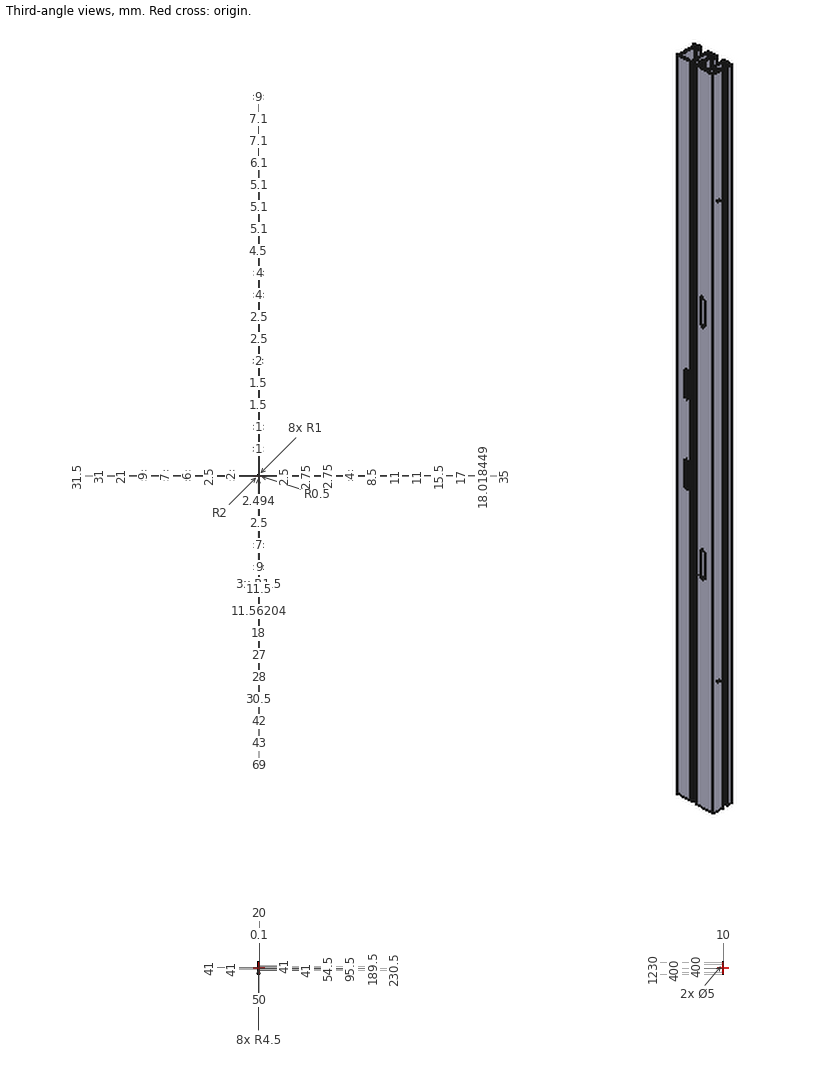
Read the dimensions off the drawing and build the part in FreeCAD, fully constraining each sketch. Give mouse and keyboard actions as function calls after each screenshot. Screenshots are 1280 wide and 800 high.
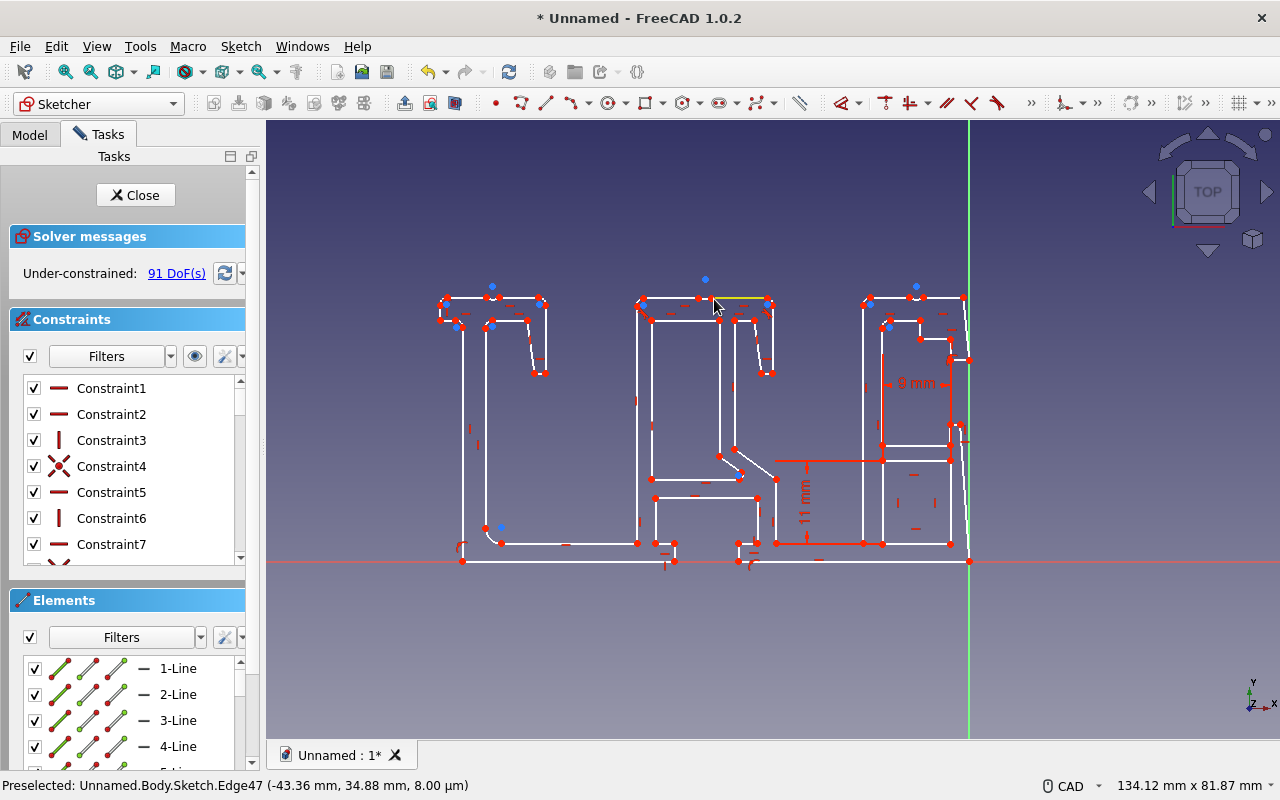
click(637, 378)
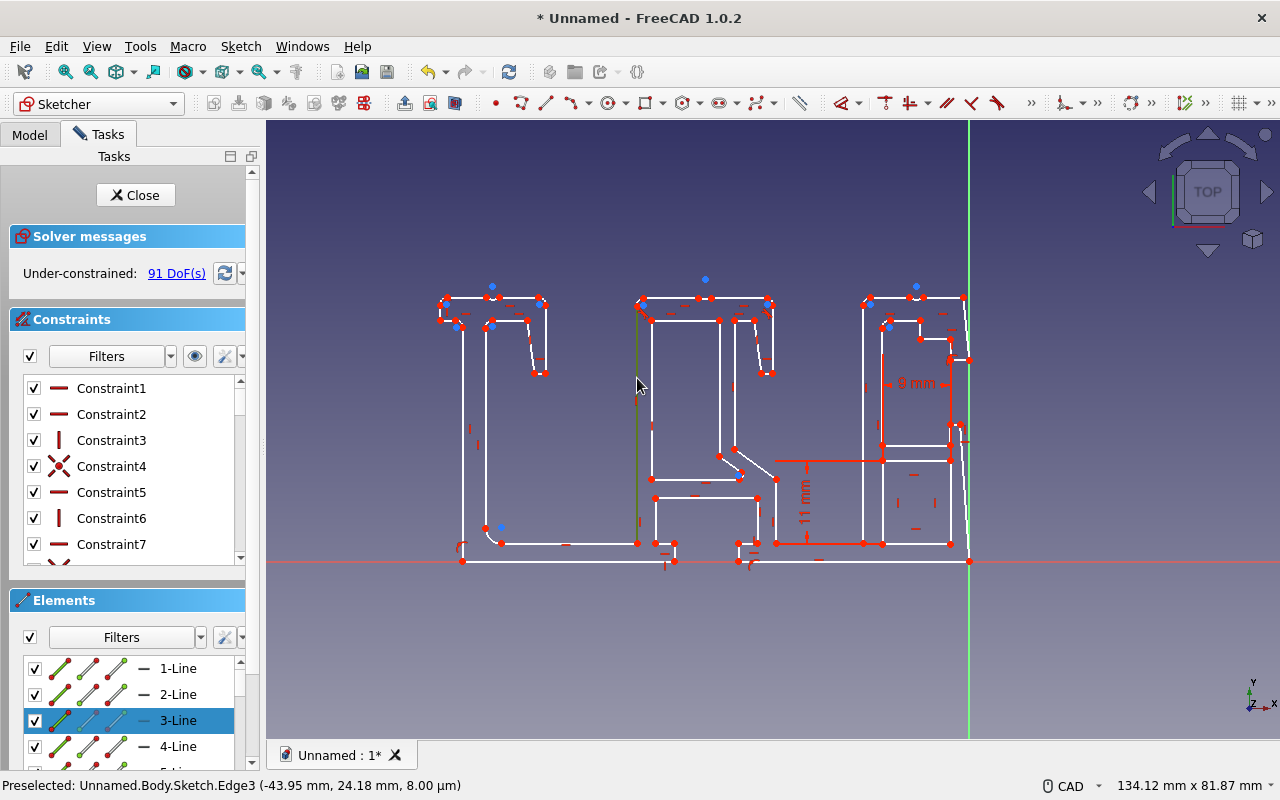
scroll(638, 301, up, 4)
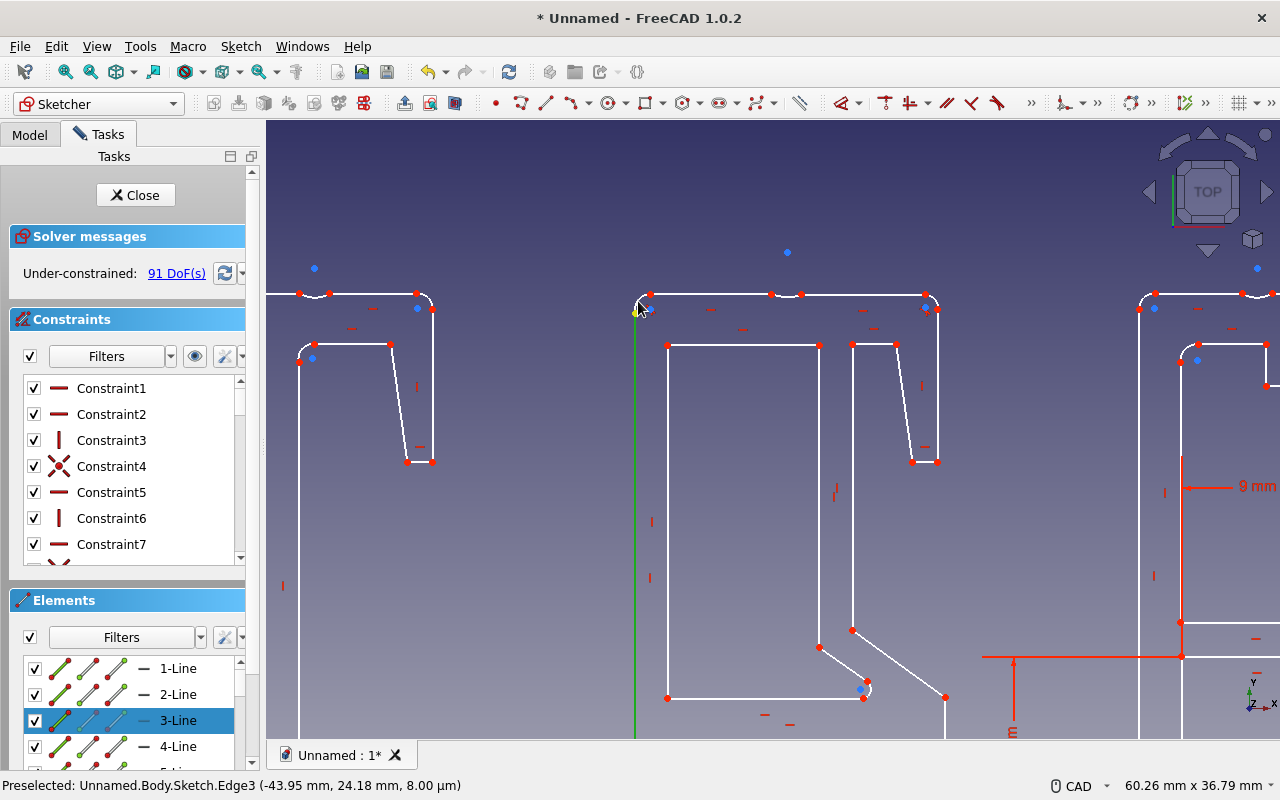
click(638, 300)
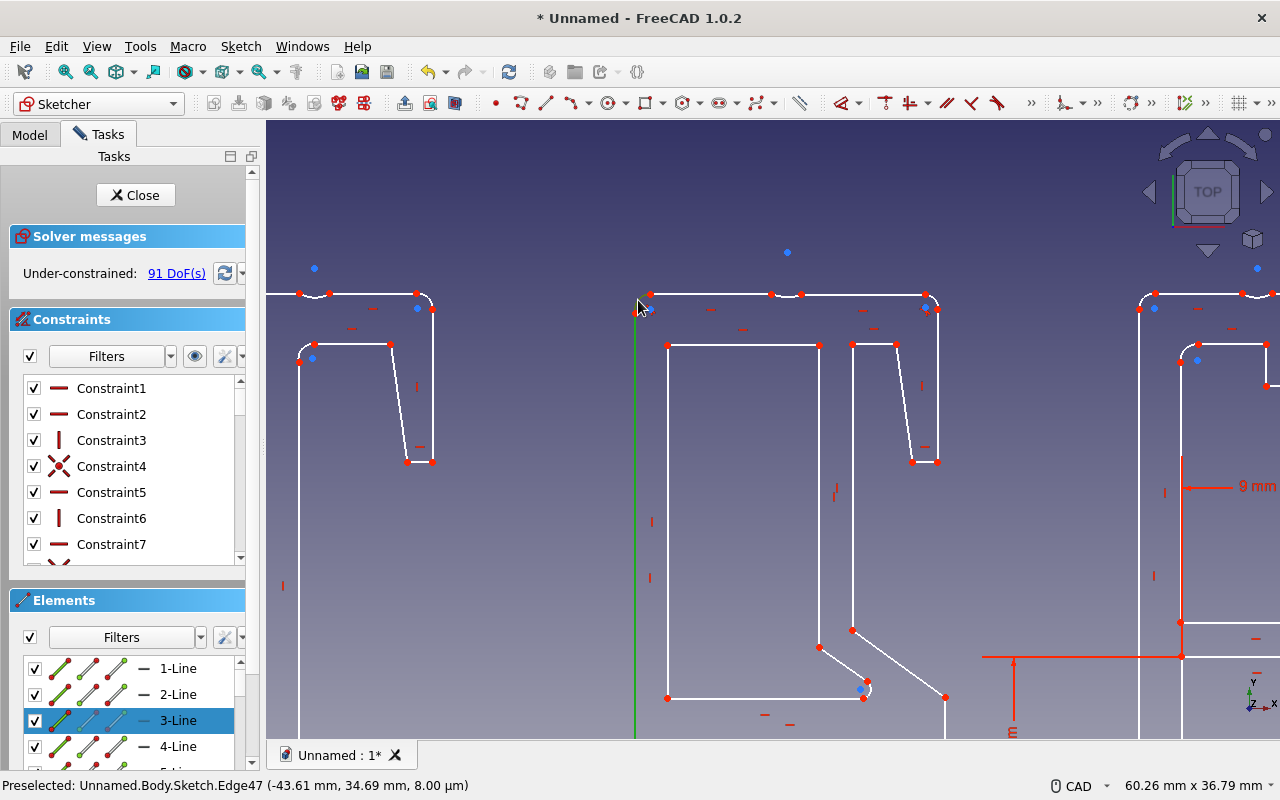
click(997, 104)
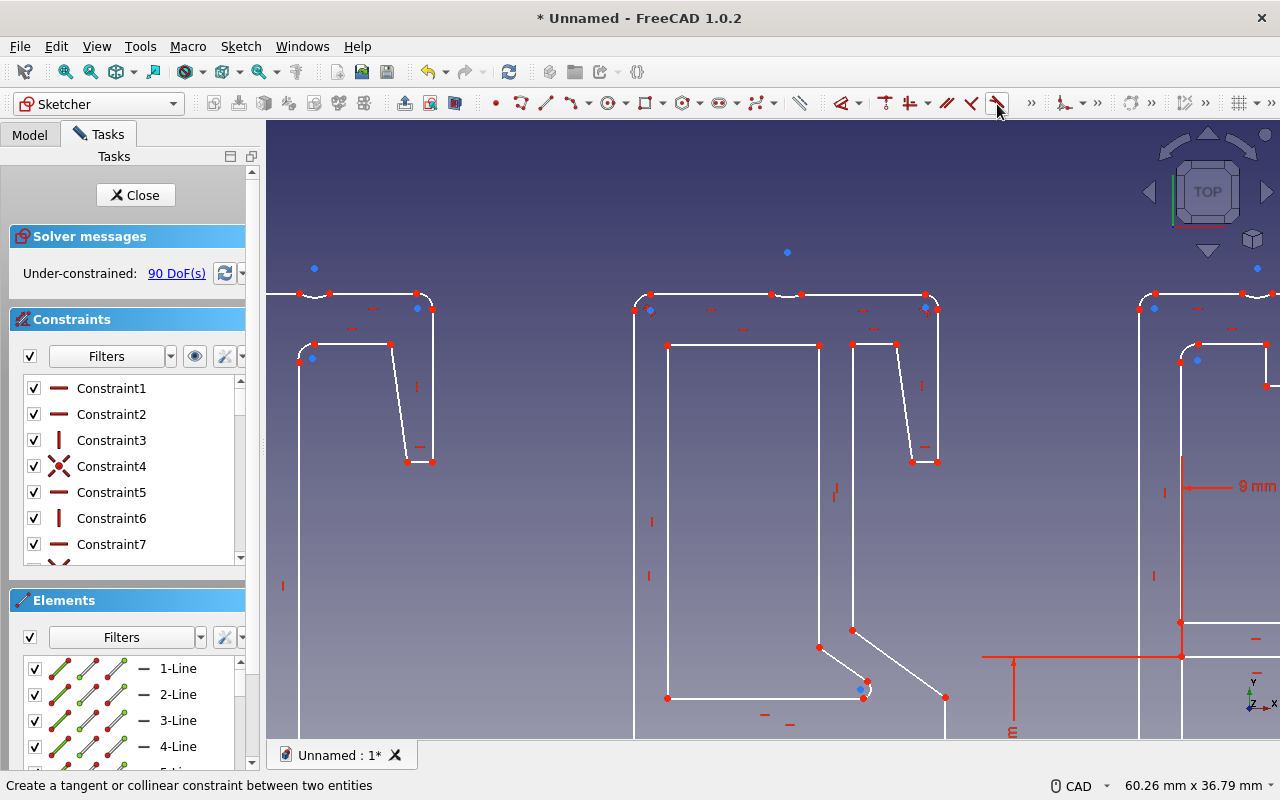
scroll(638, 301, down, 4)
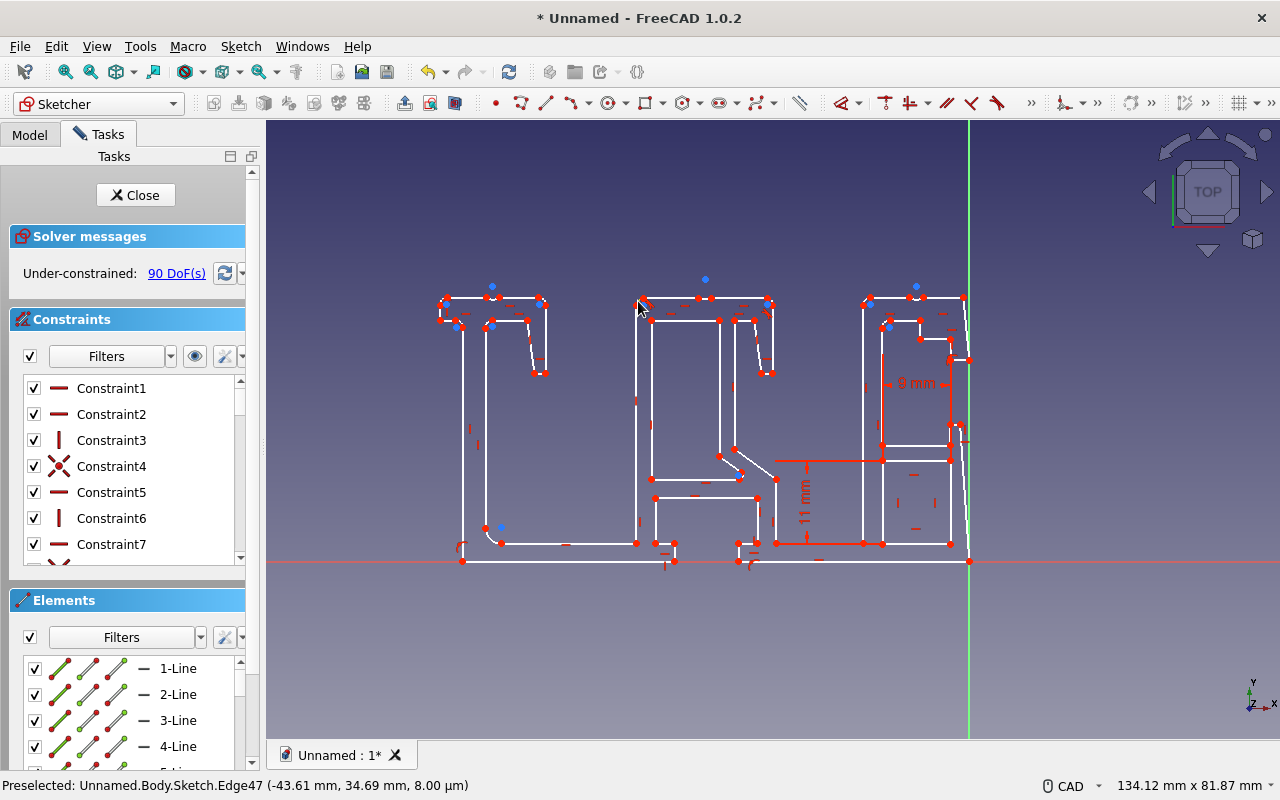
click(596, 544)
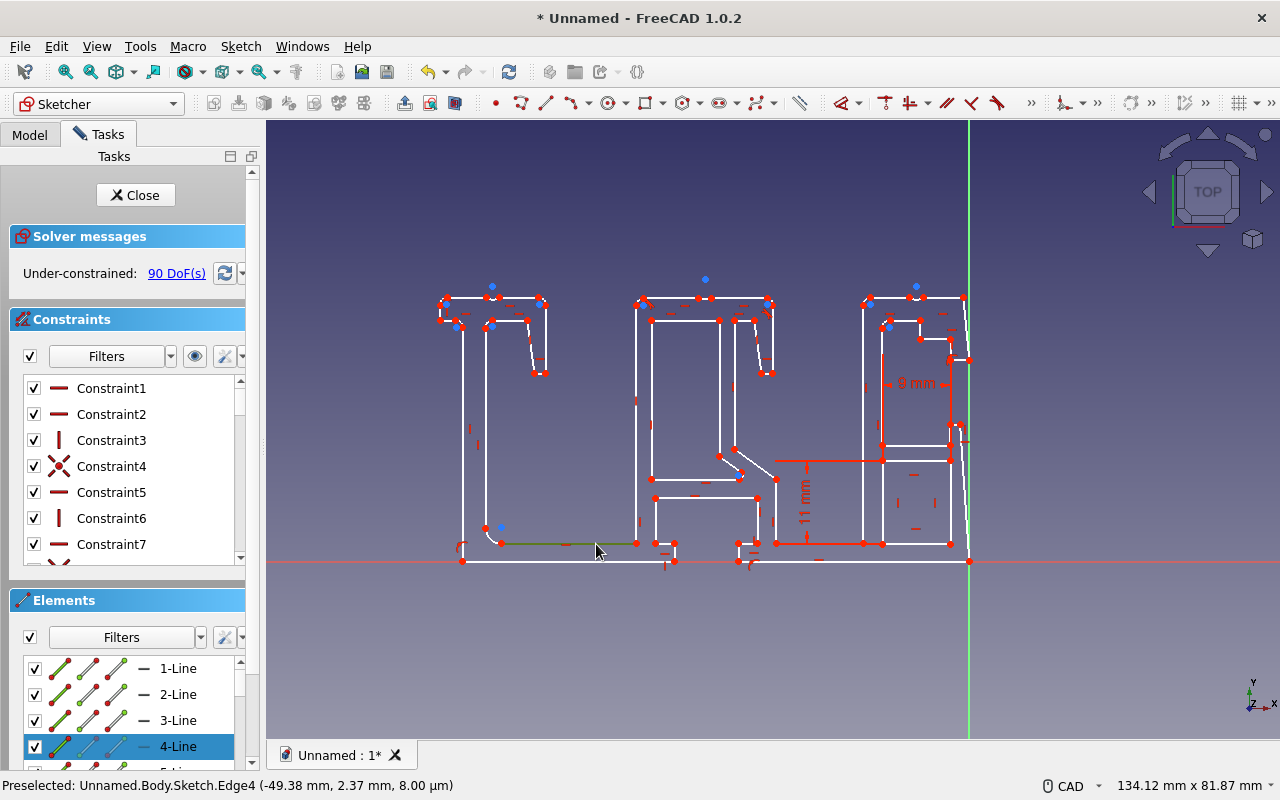
click(491, 539)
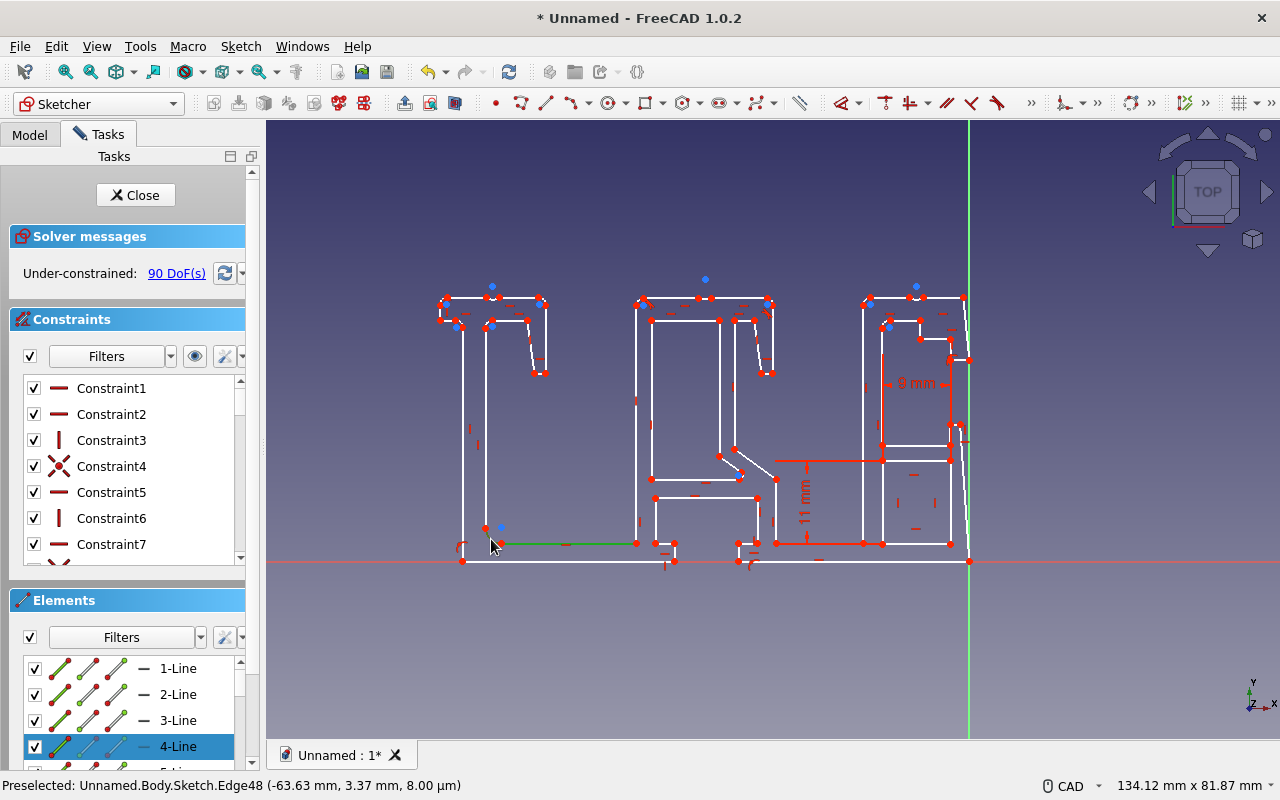
click(997, 104)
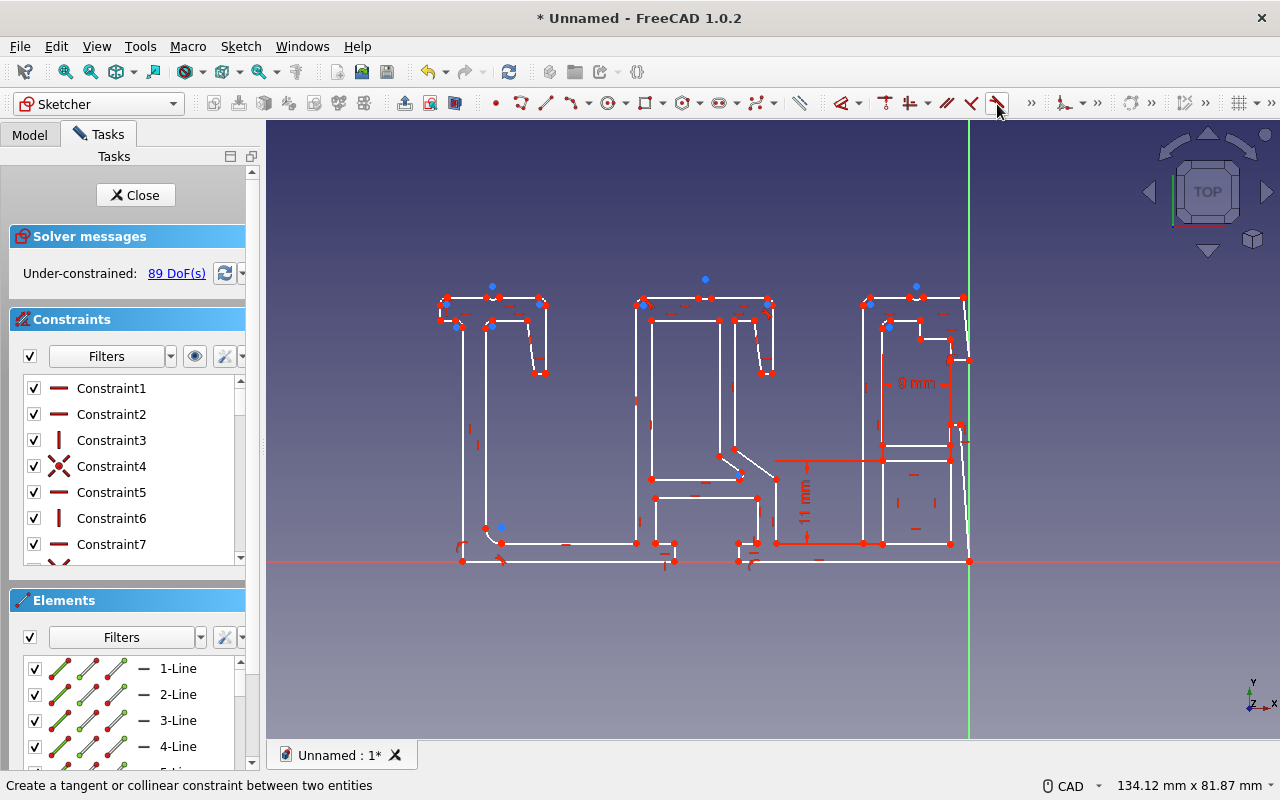
click(486, 469)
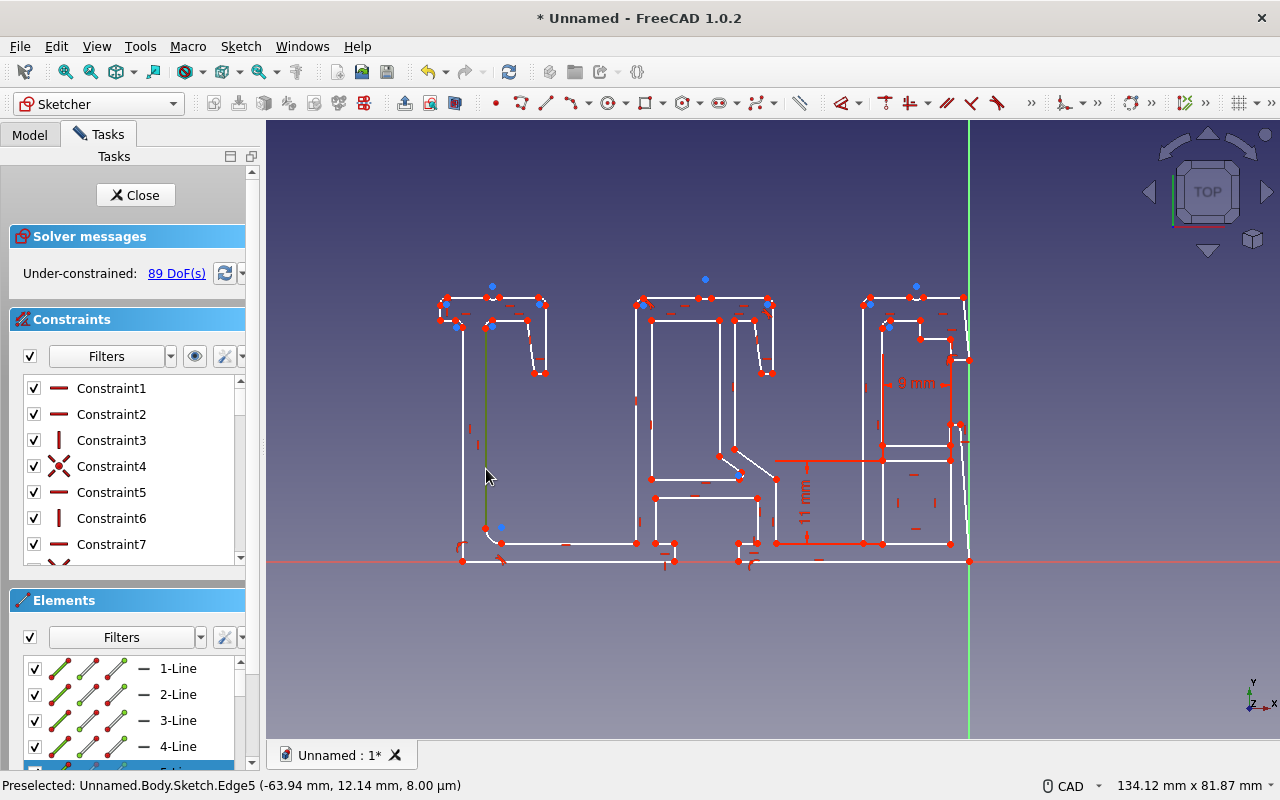
click(491, 540)